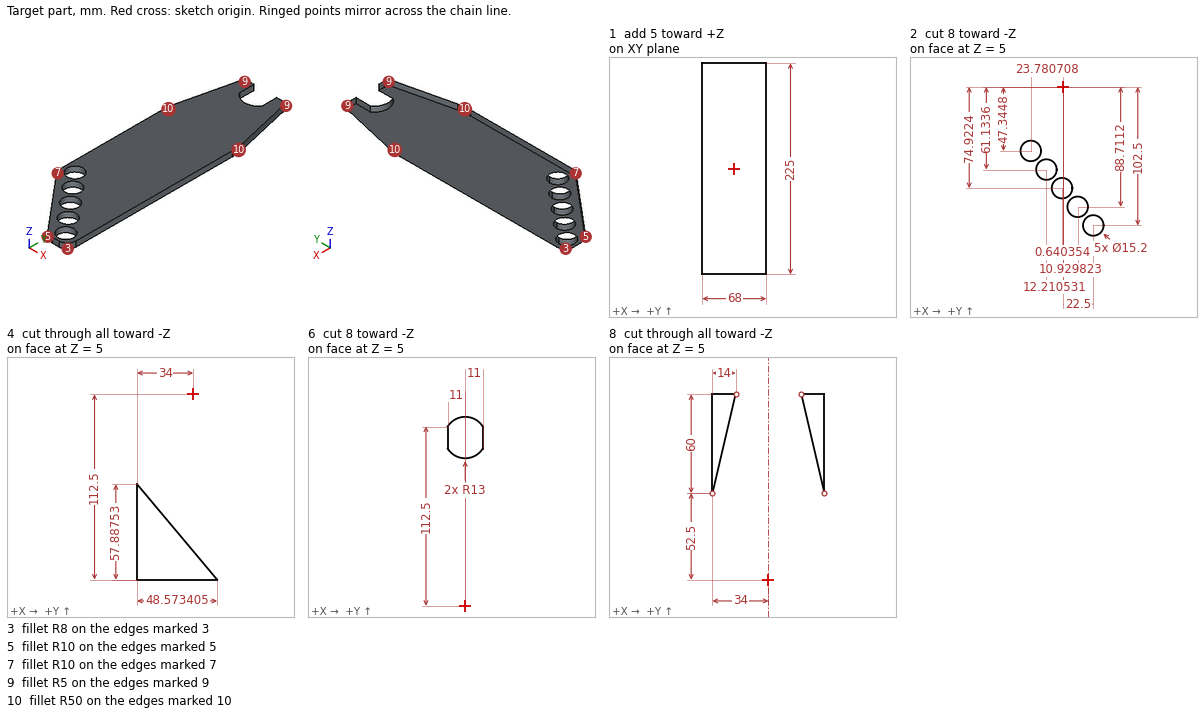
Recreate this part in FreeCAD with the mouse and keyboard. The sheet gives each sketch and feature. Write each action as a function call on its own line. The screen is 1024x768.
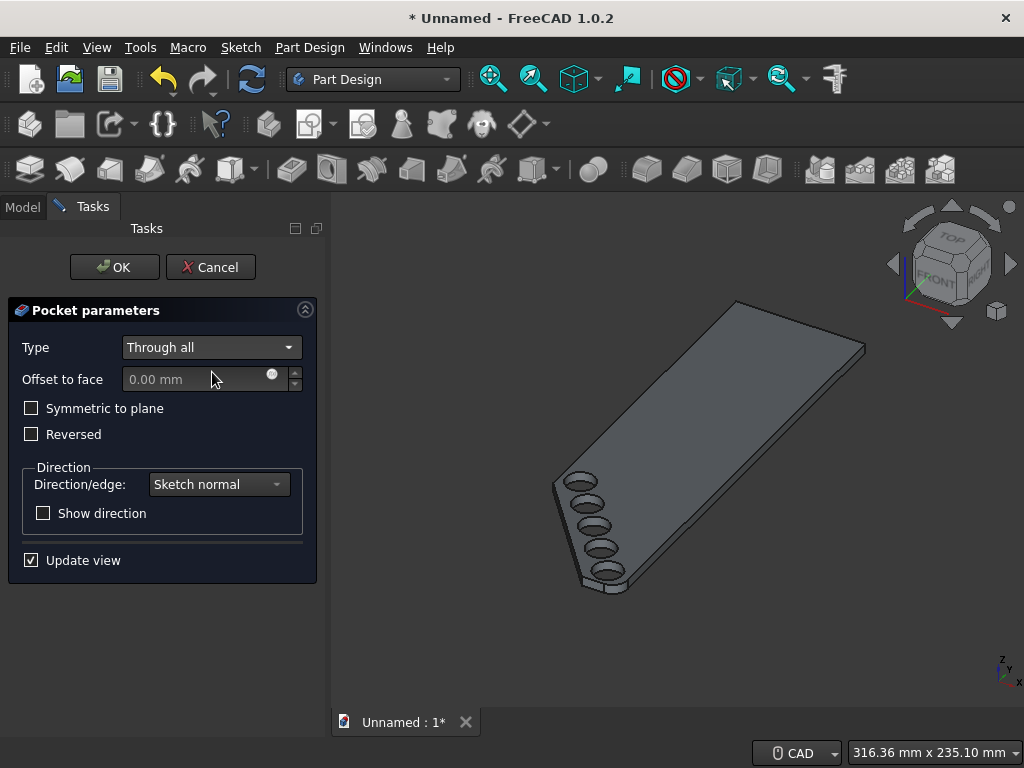
click(115, 267)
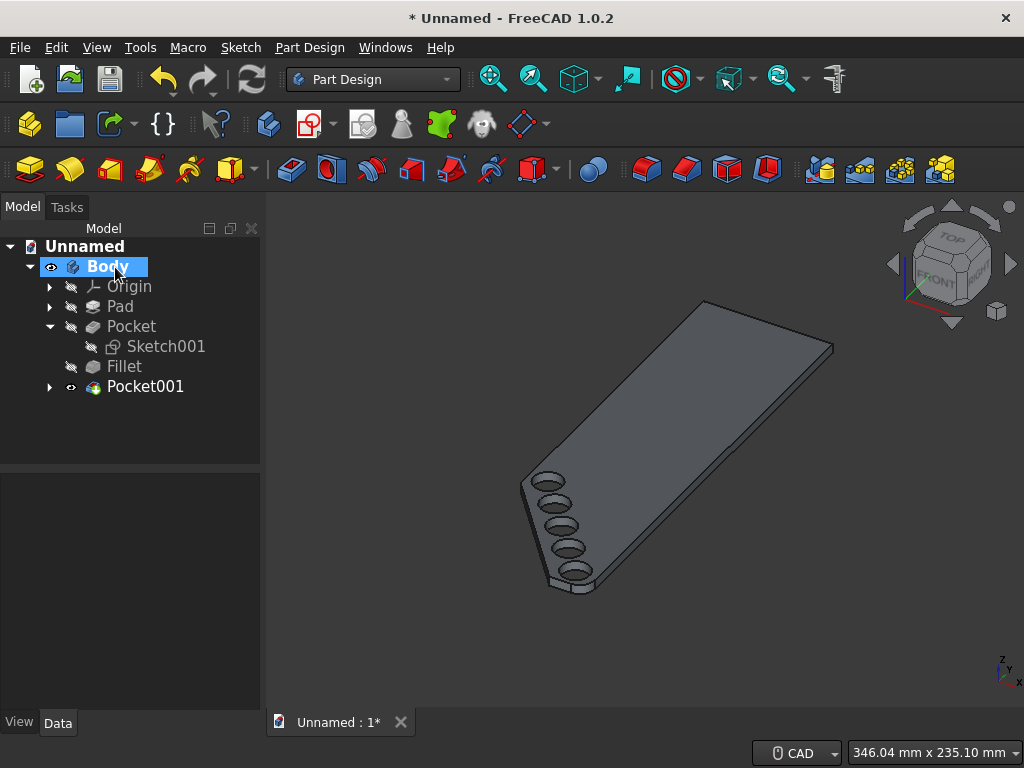
scroll(549, 580, up, 7)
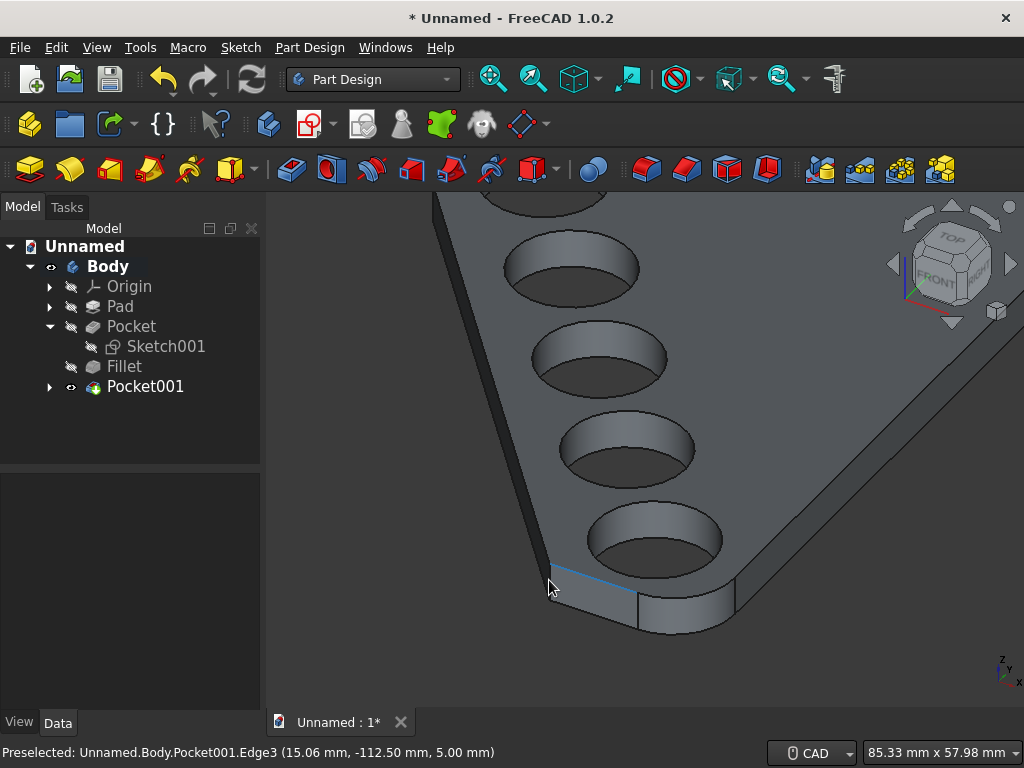
key(v)
key(f)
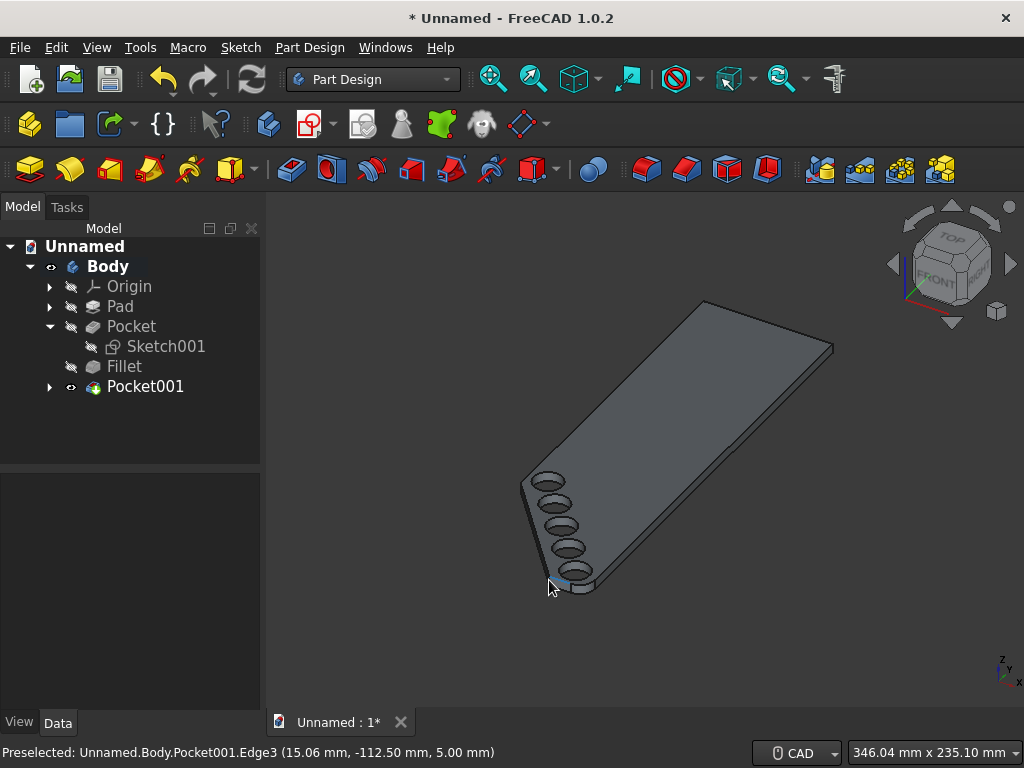
key(0)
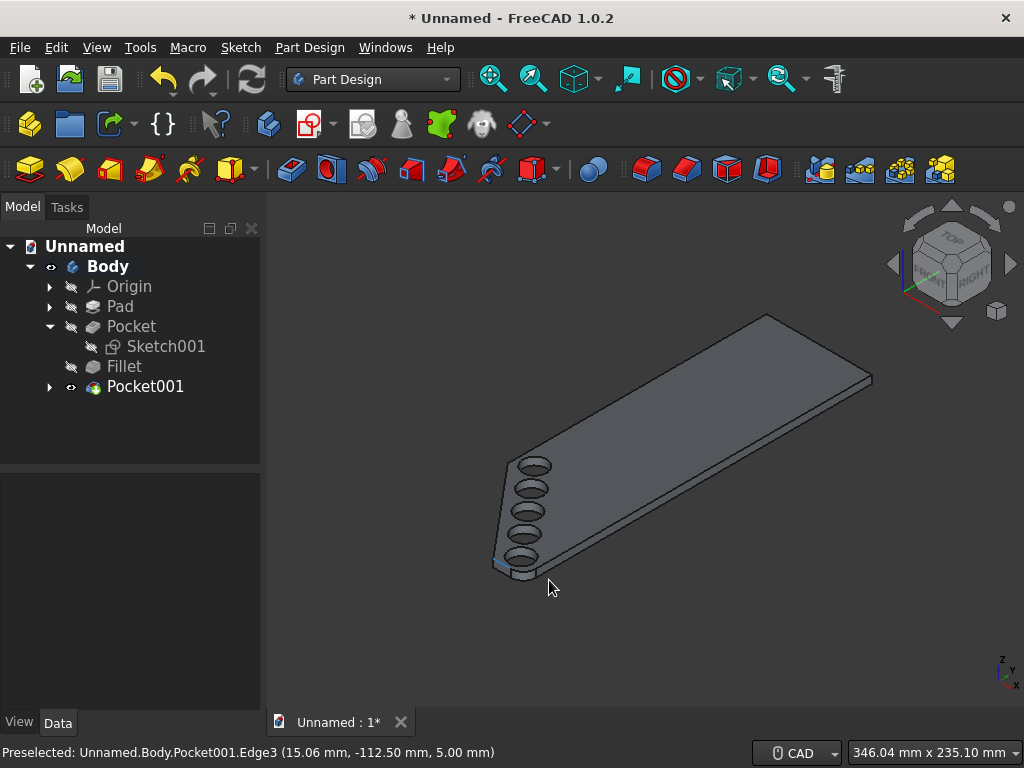
scroll(493, 562, up, 7)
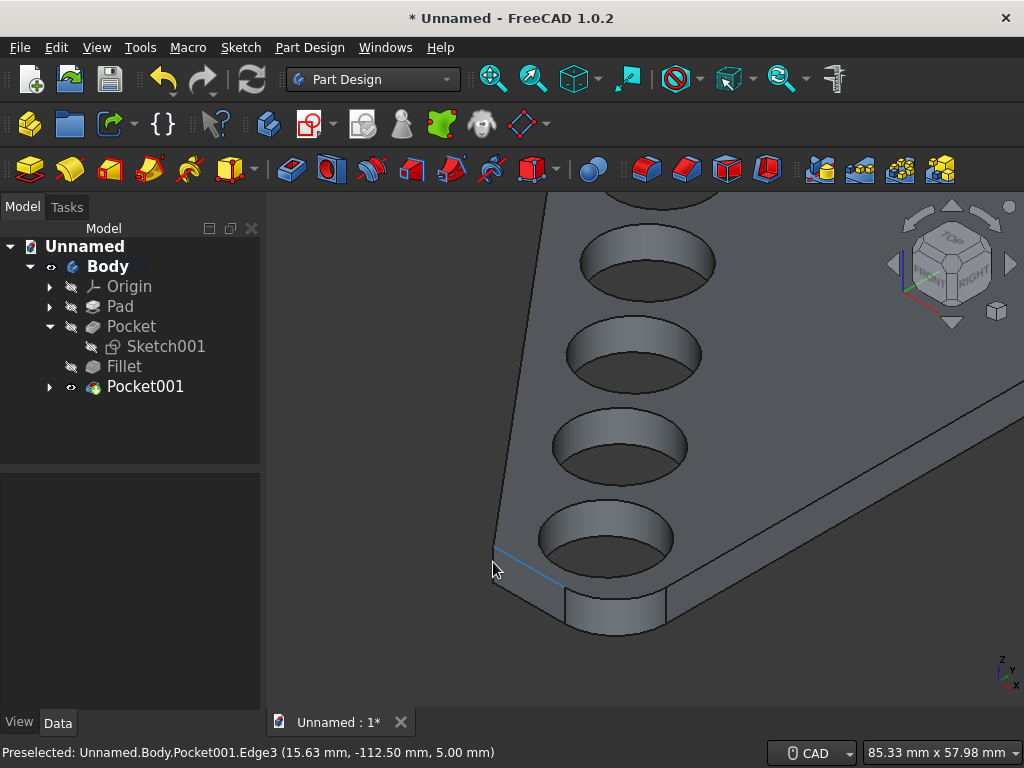
click(494, 80)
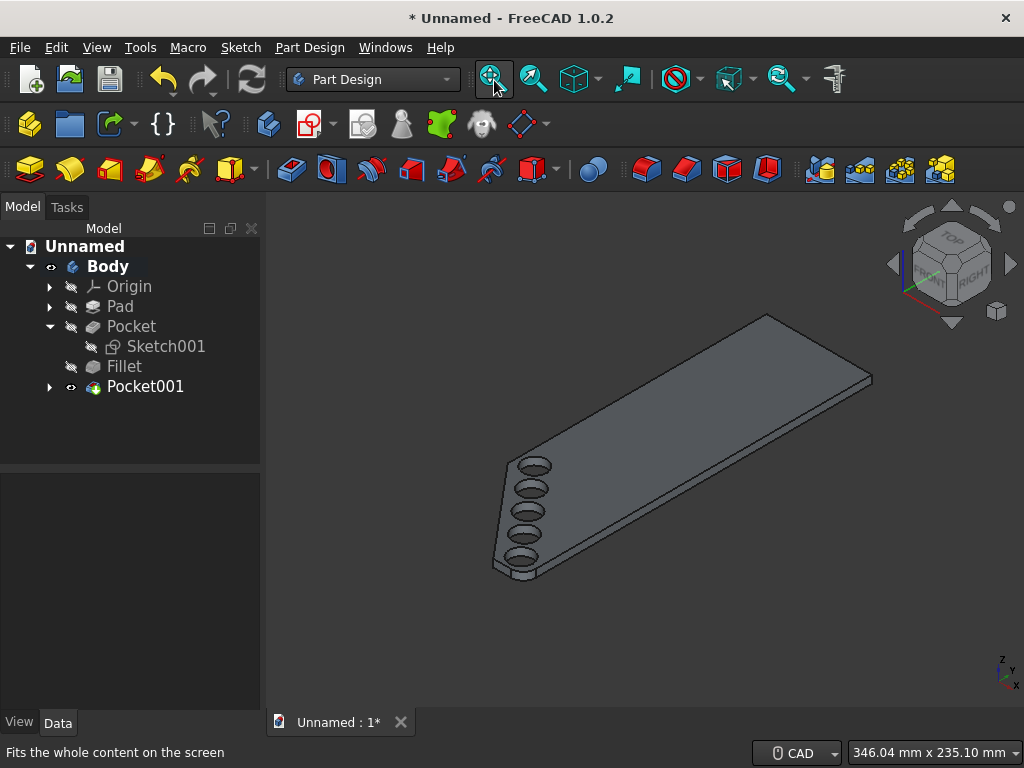
key(2)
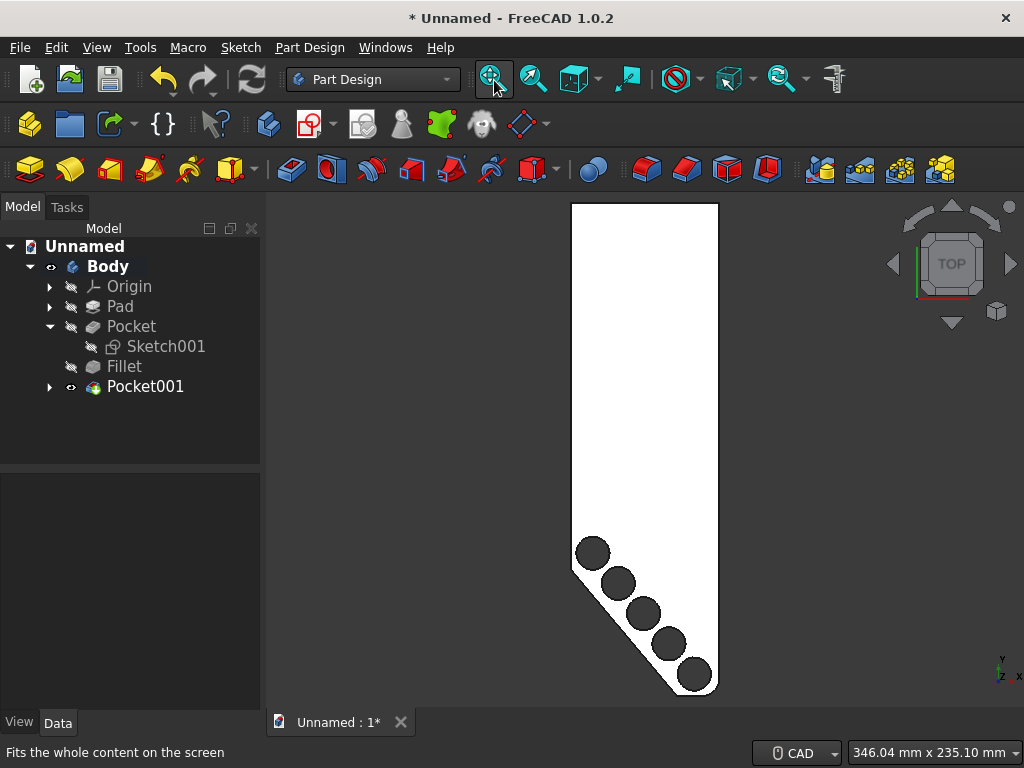
key(1)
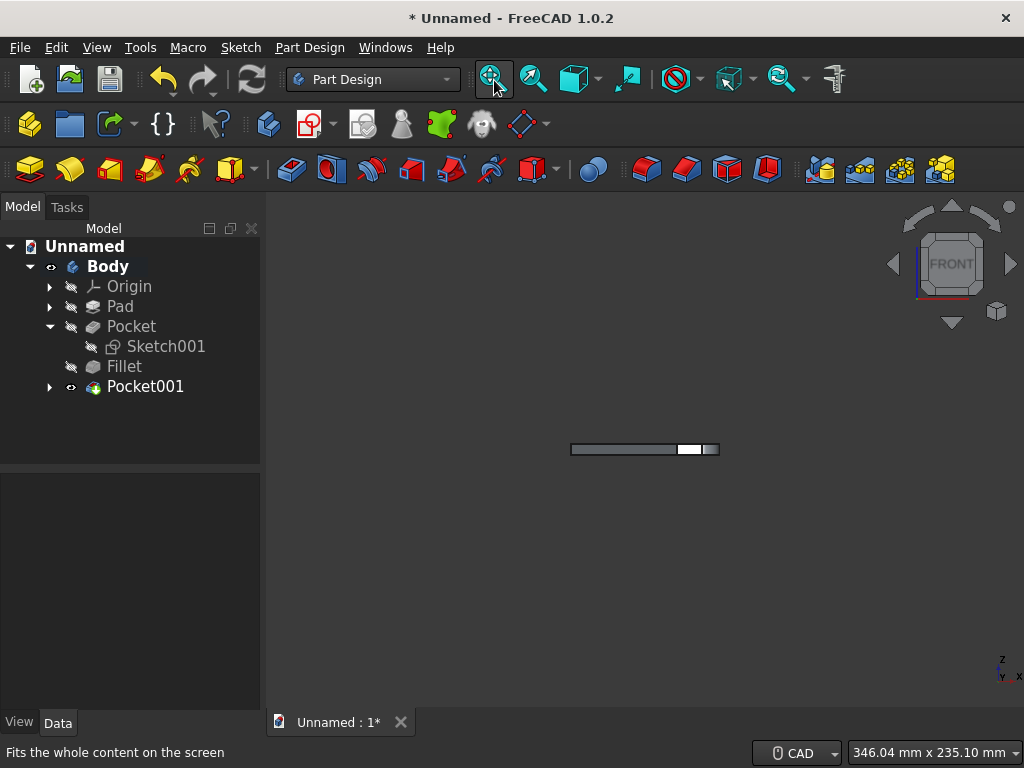
click(494, 80)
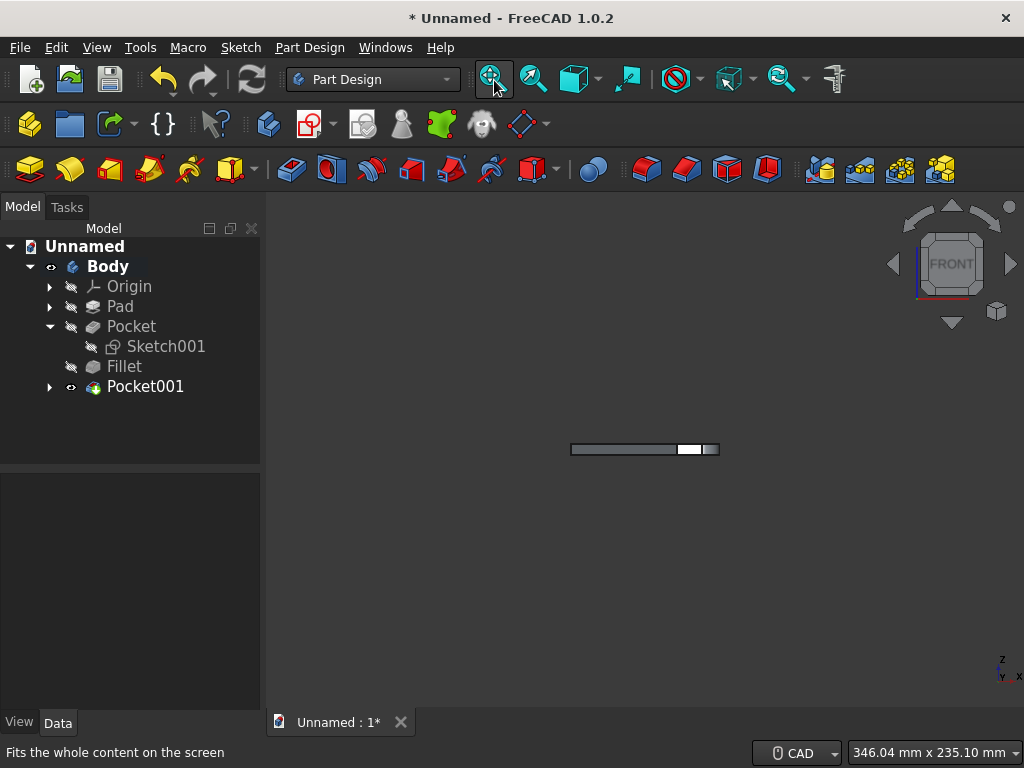
scroll(677, 449, up, 7)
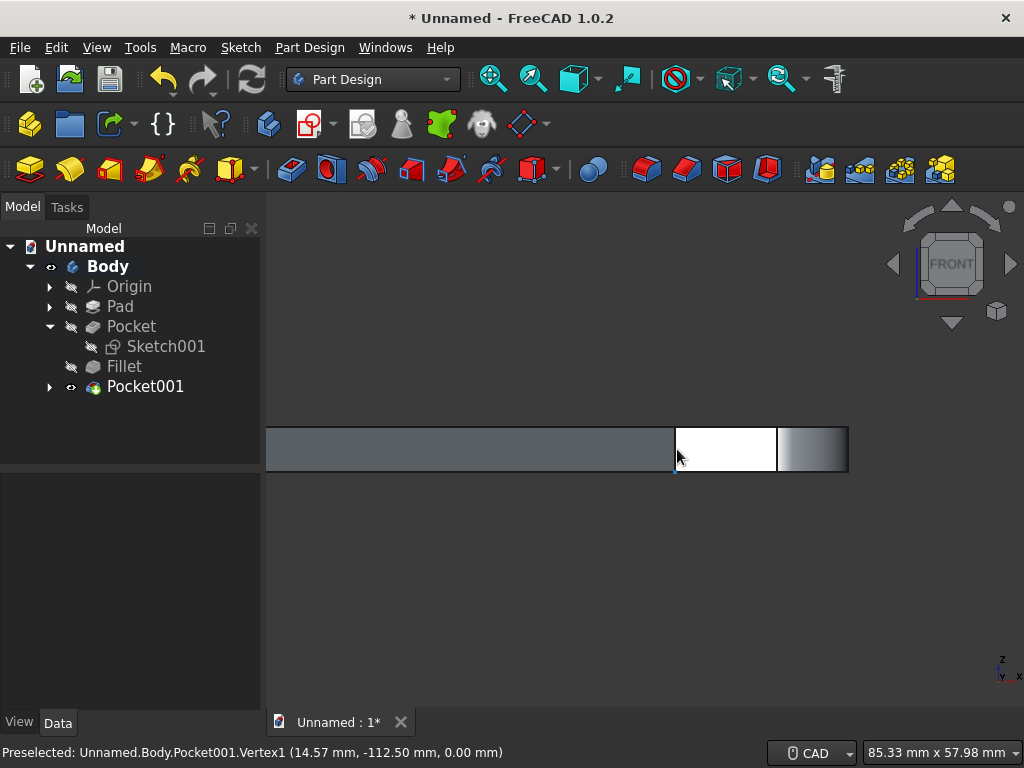
click(675, 449)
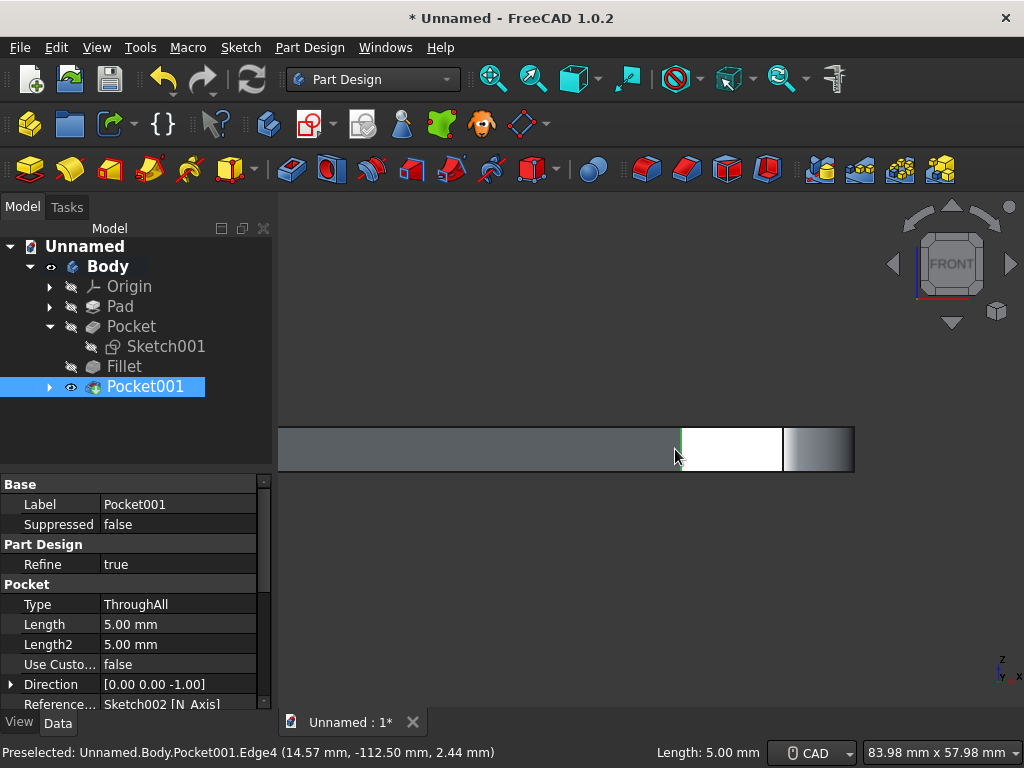
click(648, 170)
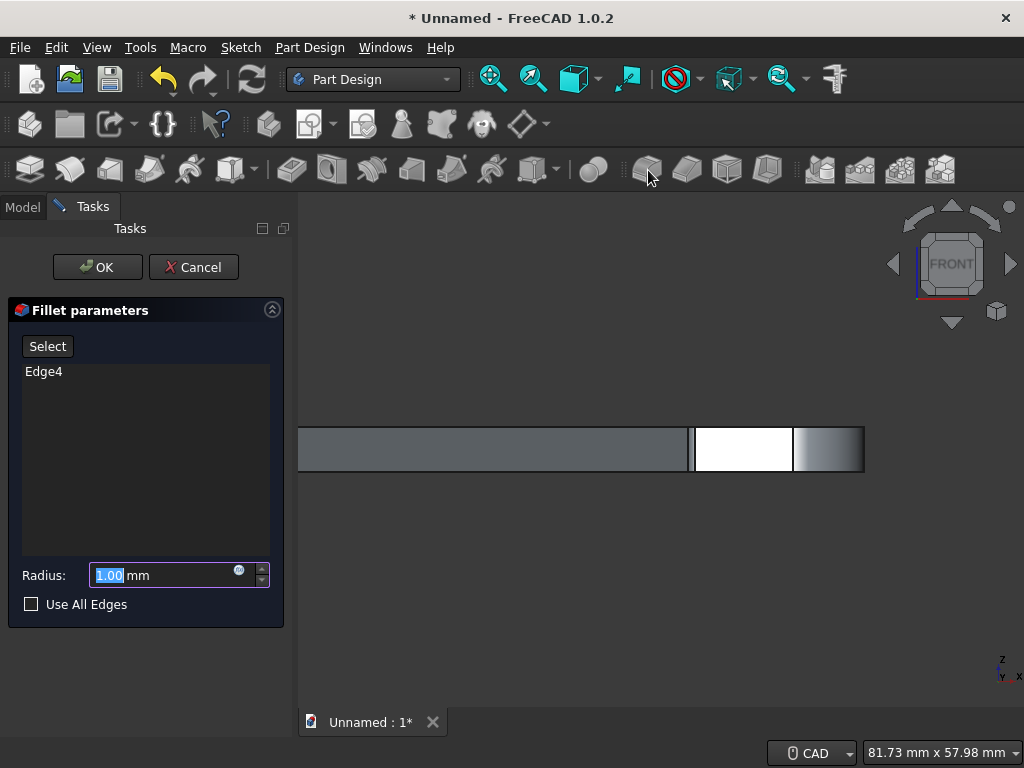
text(10)
key(Tab)